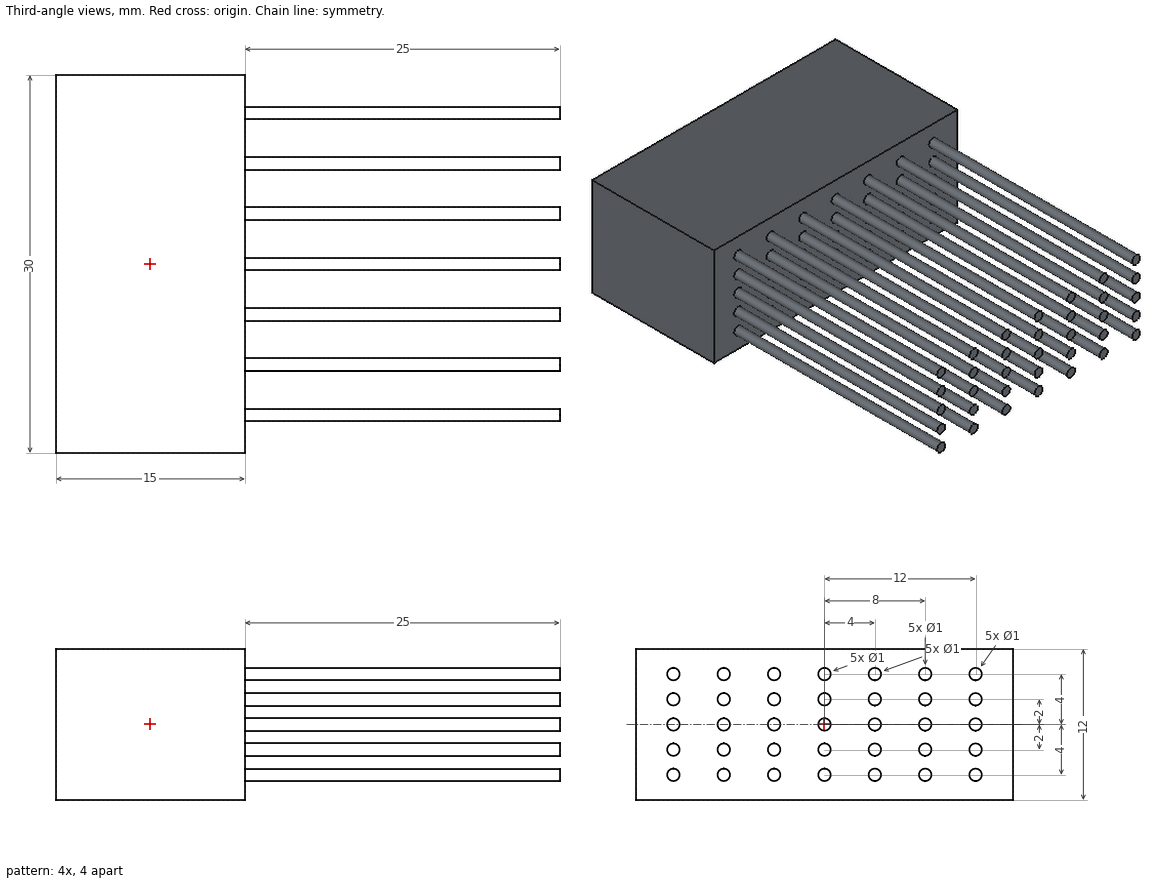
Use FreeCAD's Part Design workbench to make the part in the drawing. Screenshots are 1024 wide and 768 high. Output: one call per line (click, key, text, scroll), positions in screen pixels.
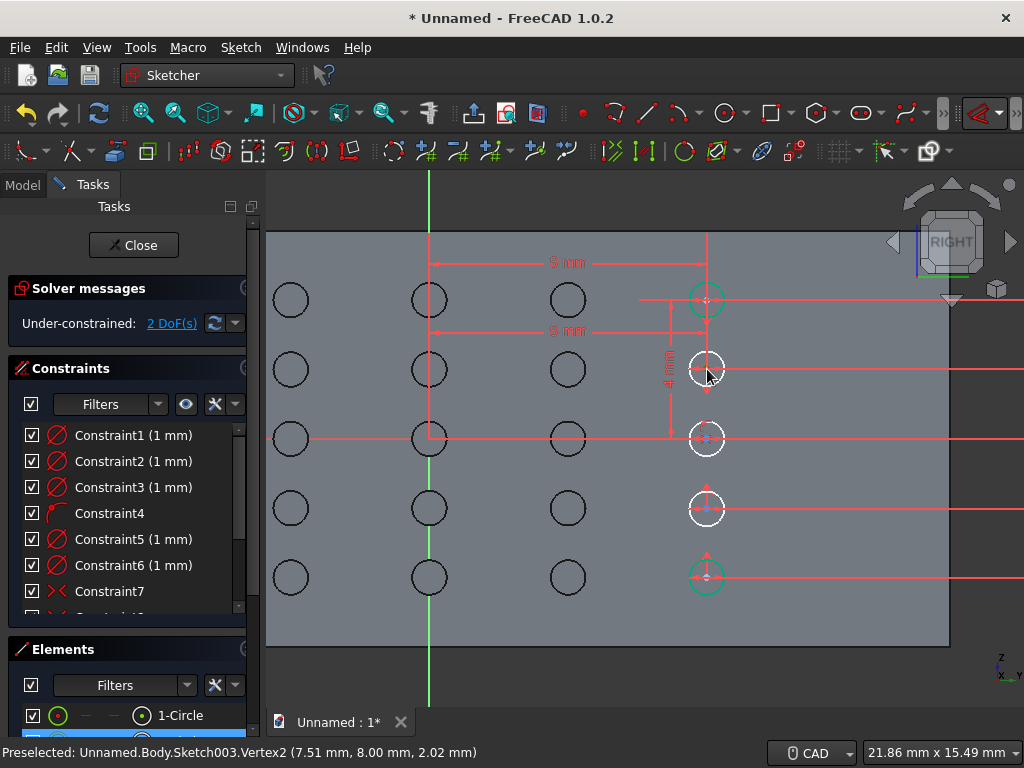
key(i)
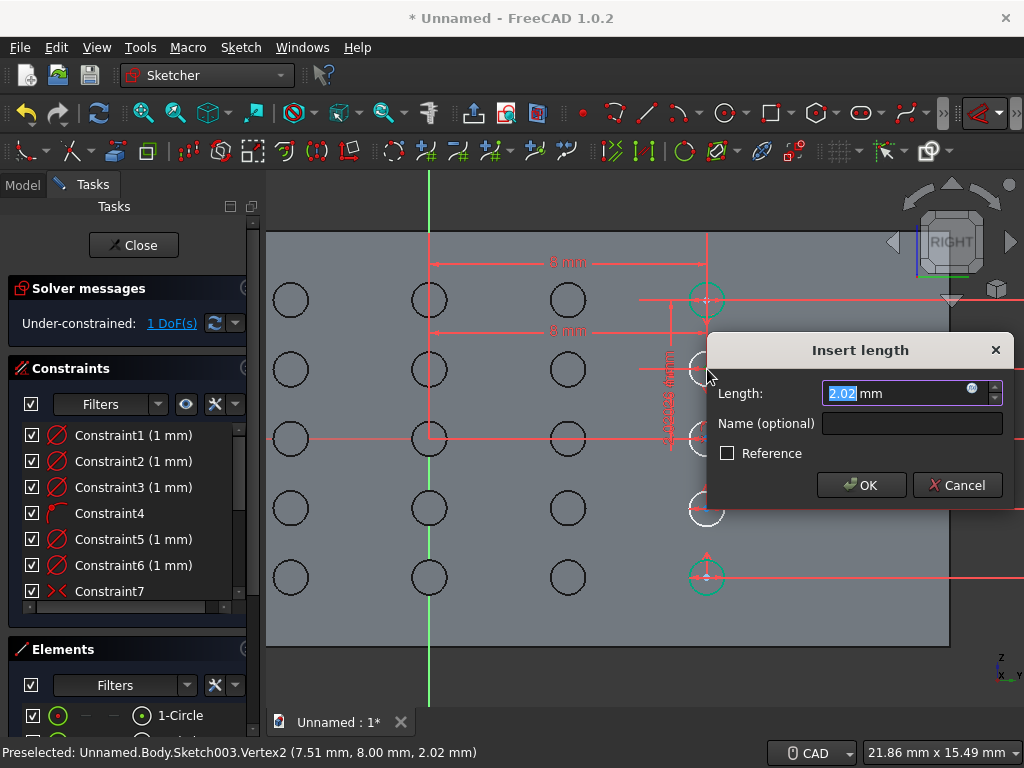
text(2)
key(Return)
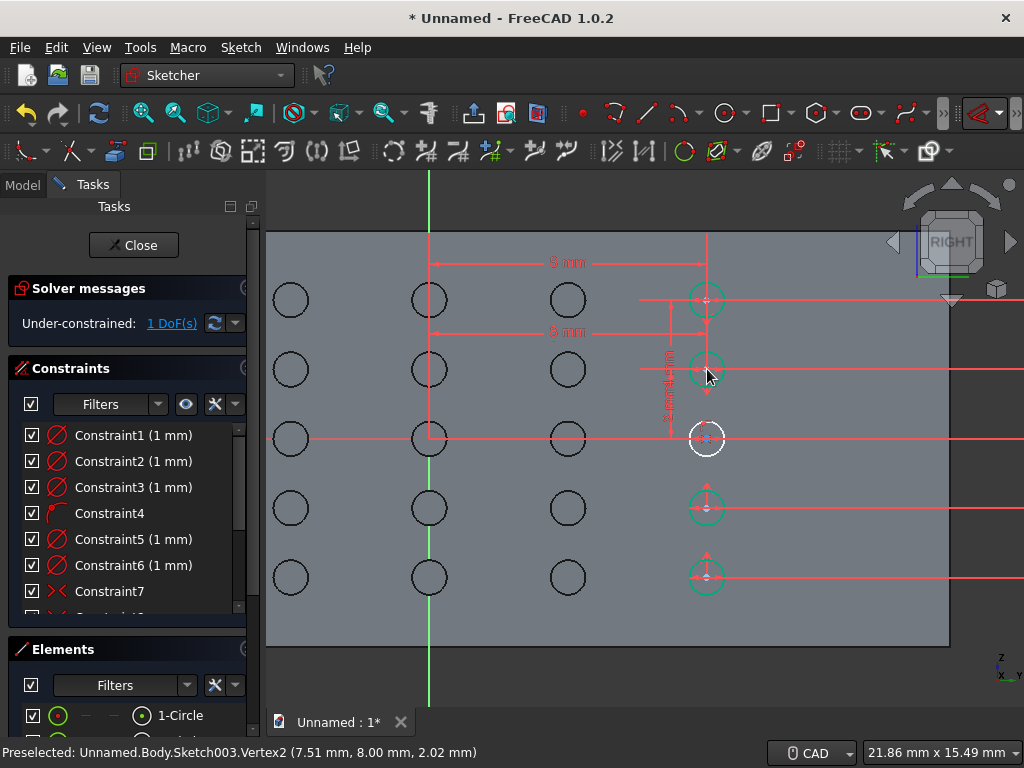
click(707, 439)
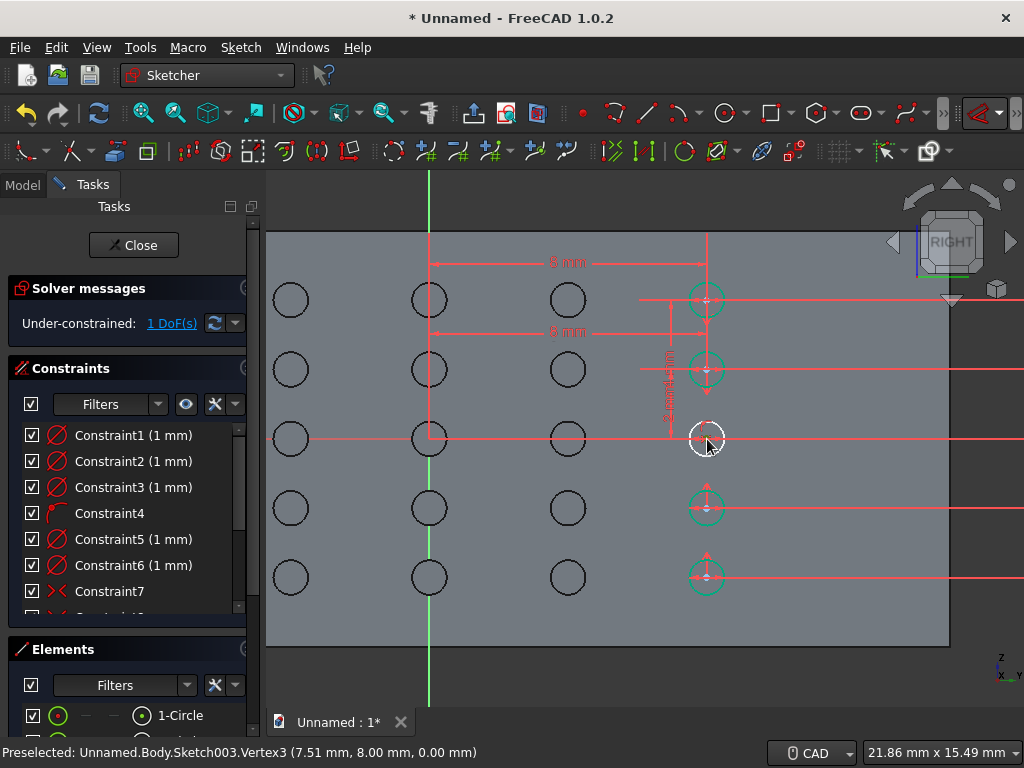
key(l)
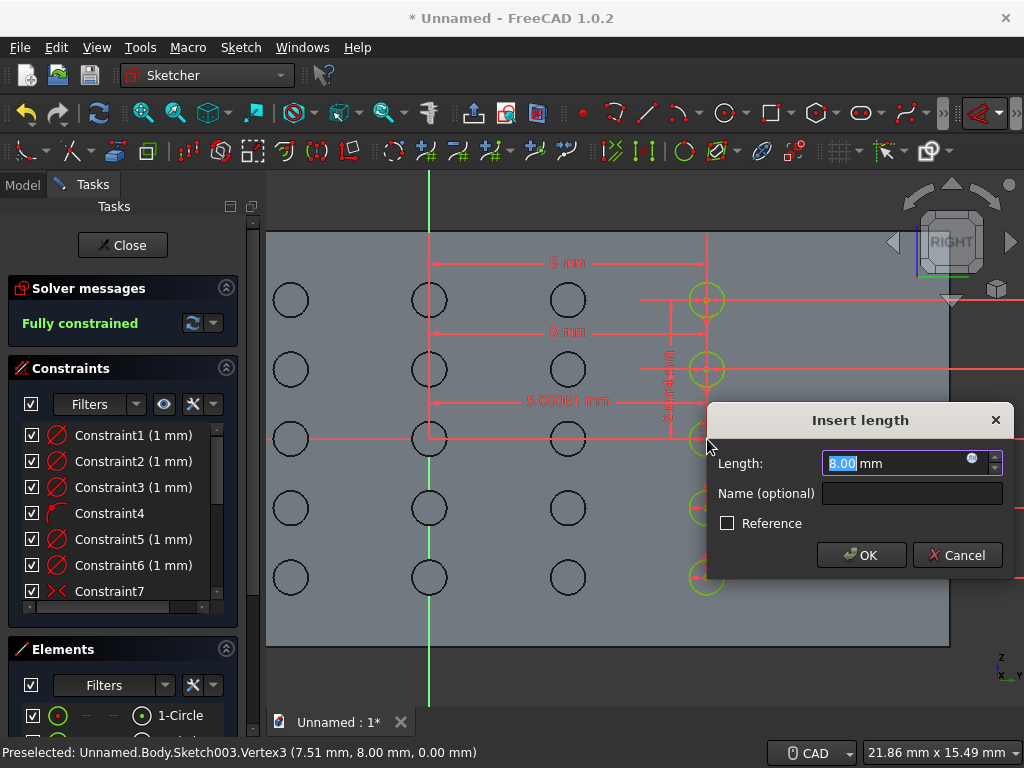
text(8)
key(Return)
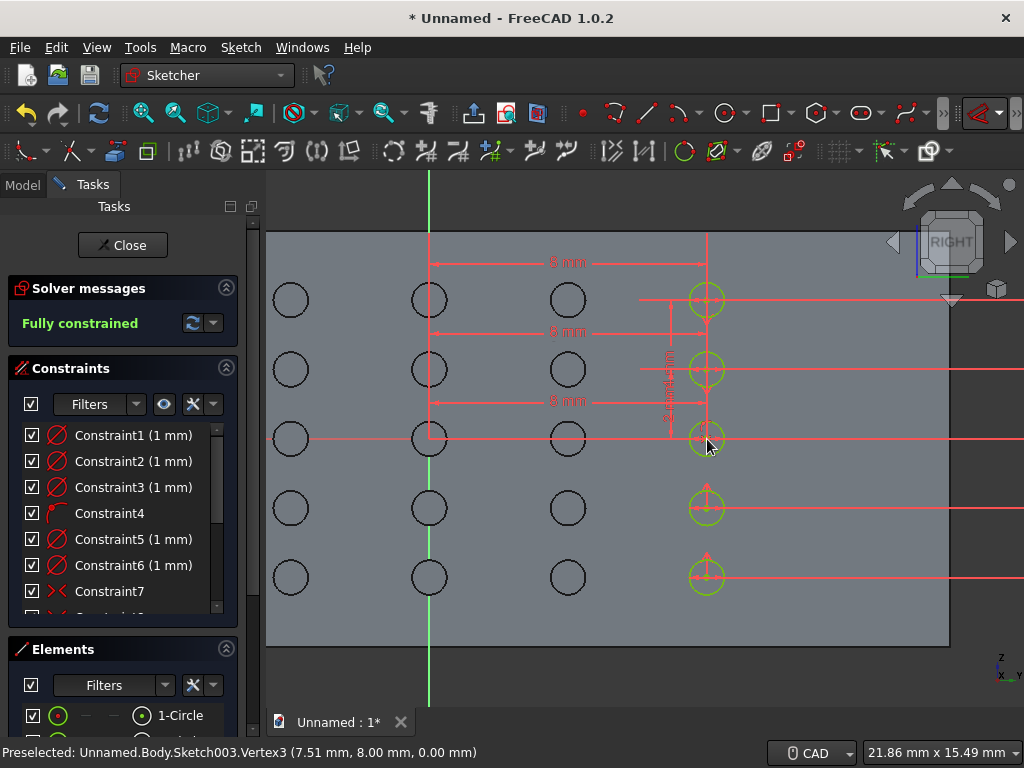
click(123, 245)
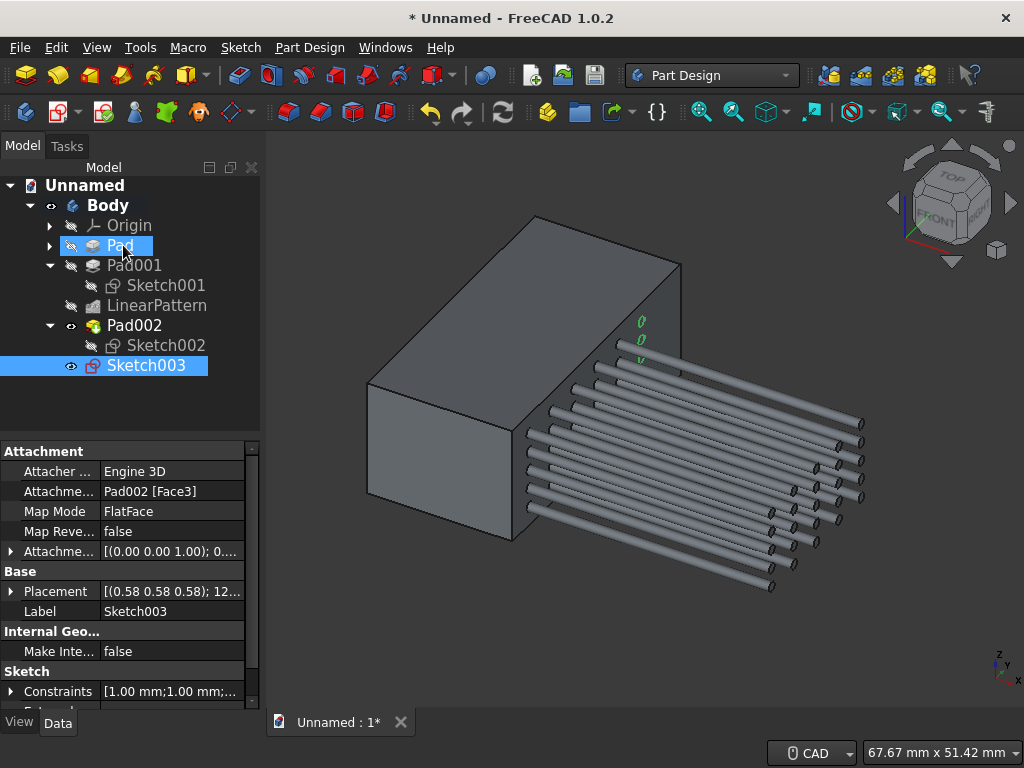
click(26, 76)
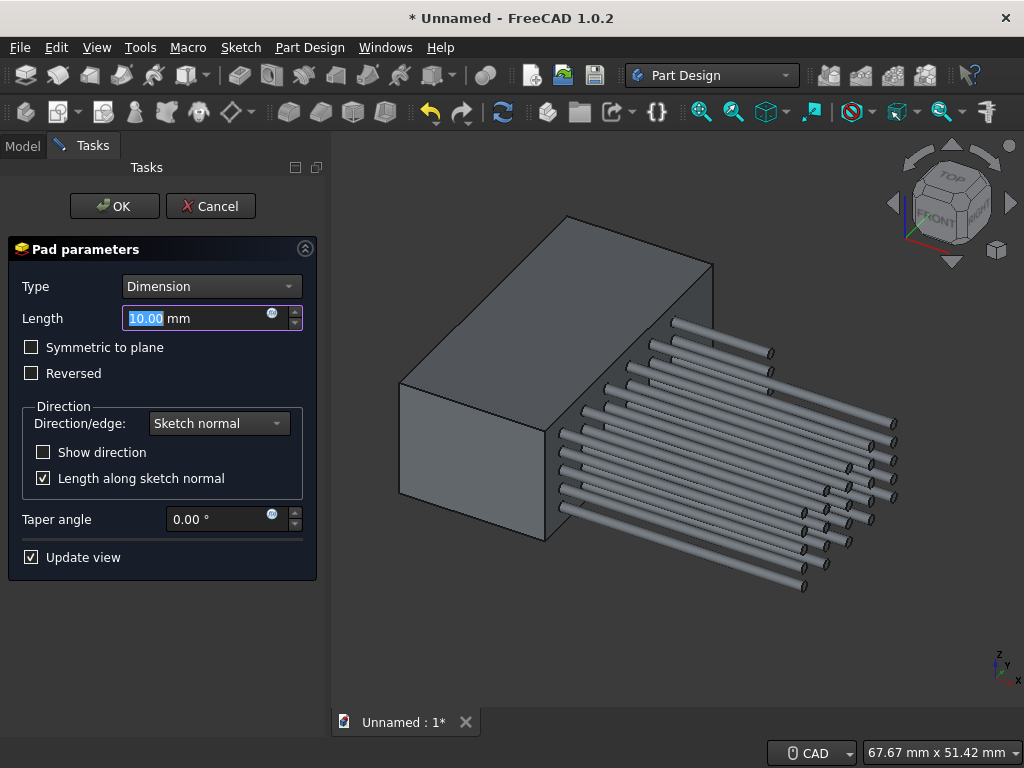
text(25)
key(Tab)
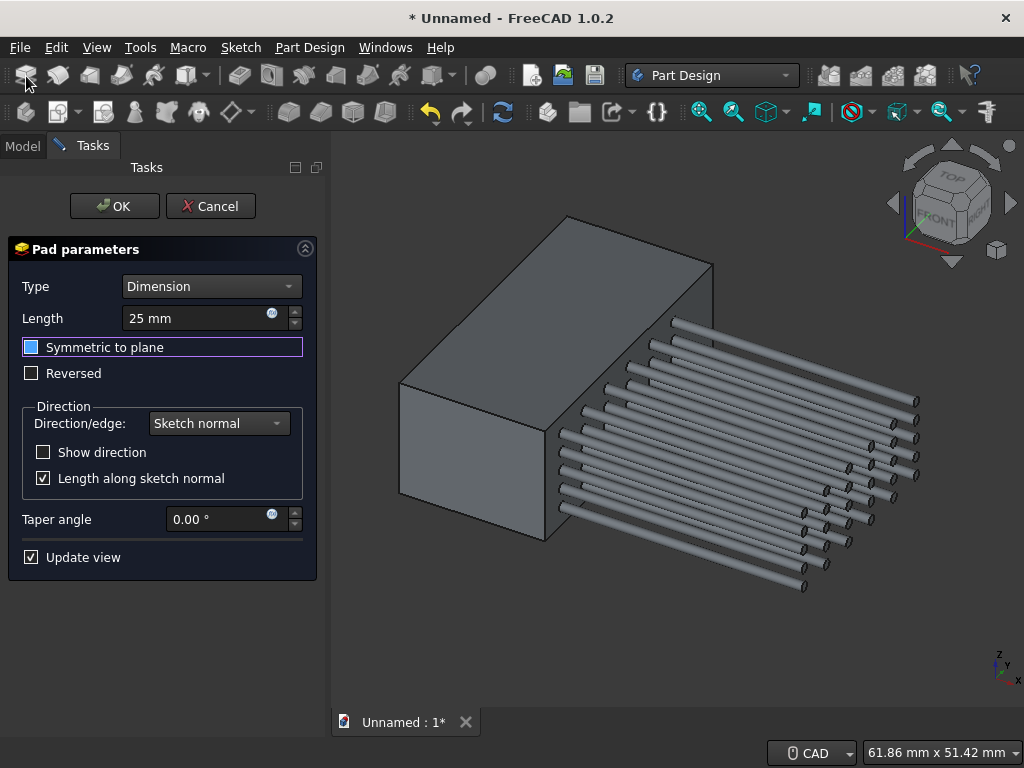
click(115, 206)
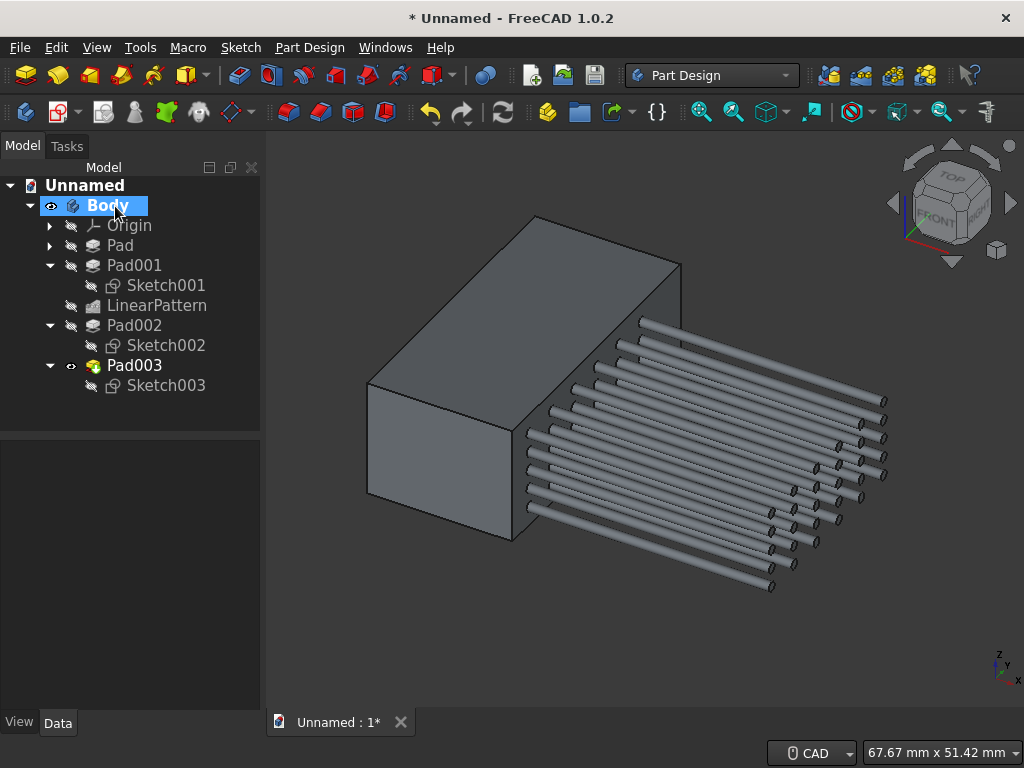
click(669, 299)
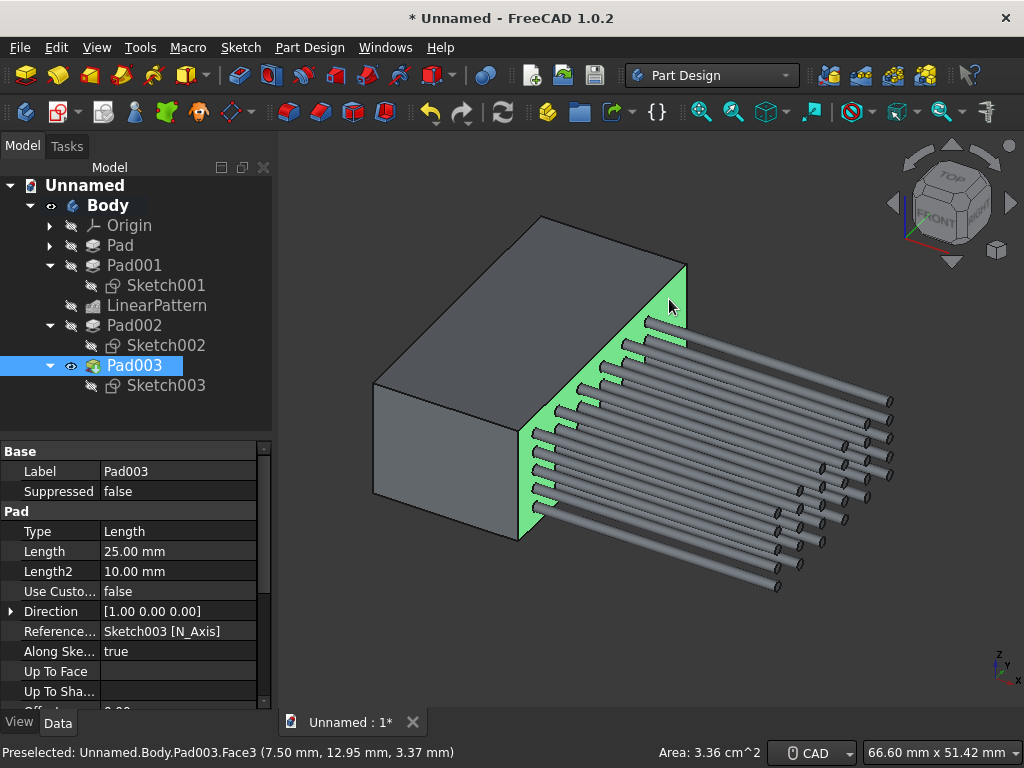
click(58, 112)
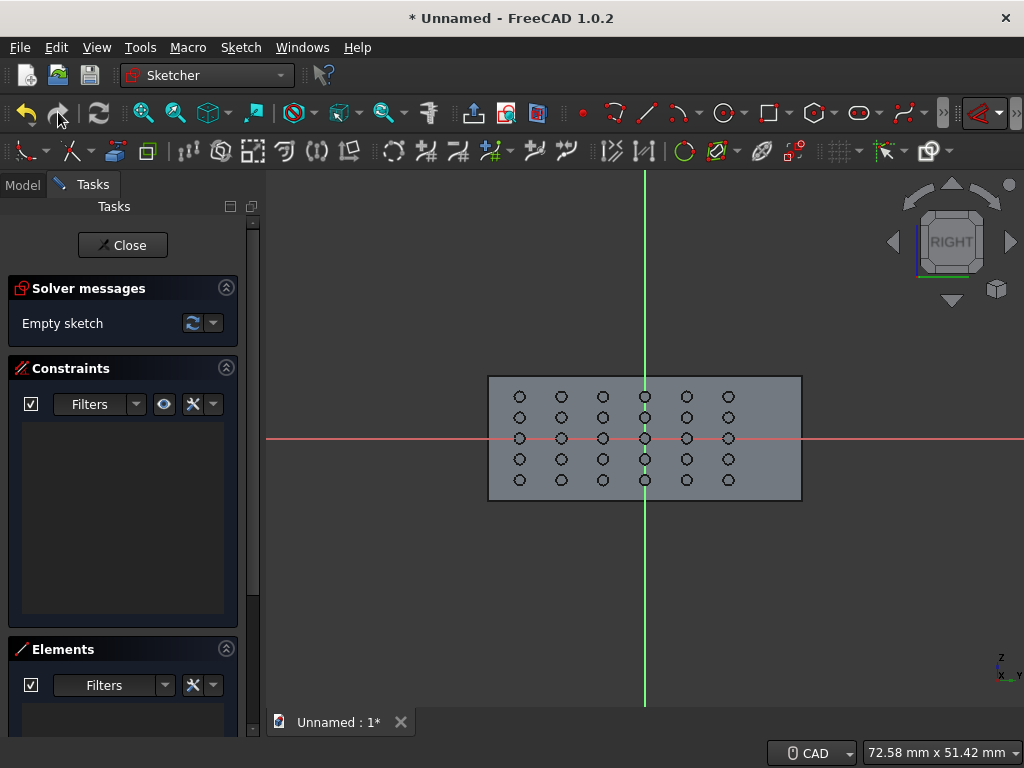
scroll(768, 438, up, 6)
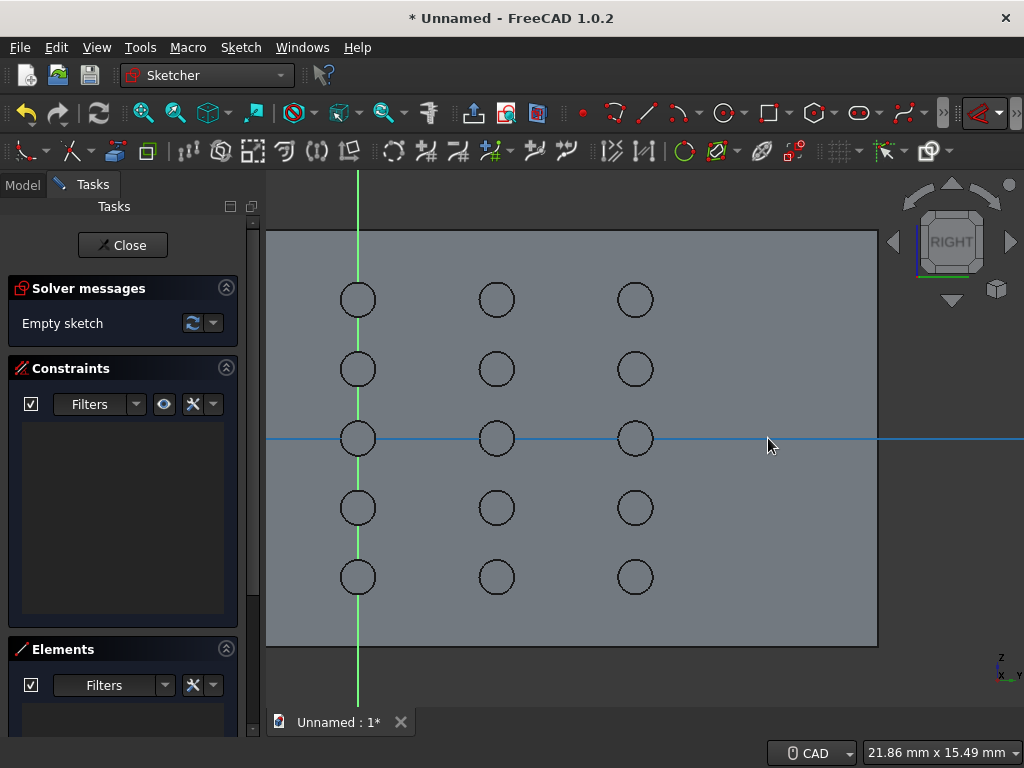
key(g)
key(c)